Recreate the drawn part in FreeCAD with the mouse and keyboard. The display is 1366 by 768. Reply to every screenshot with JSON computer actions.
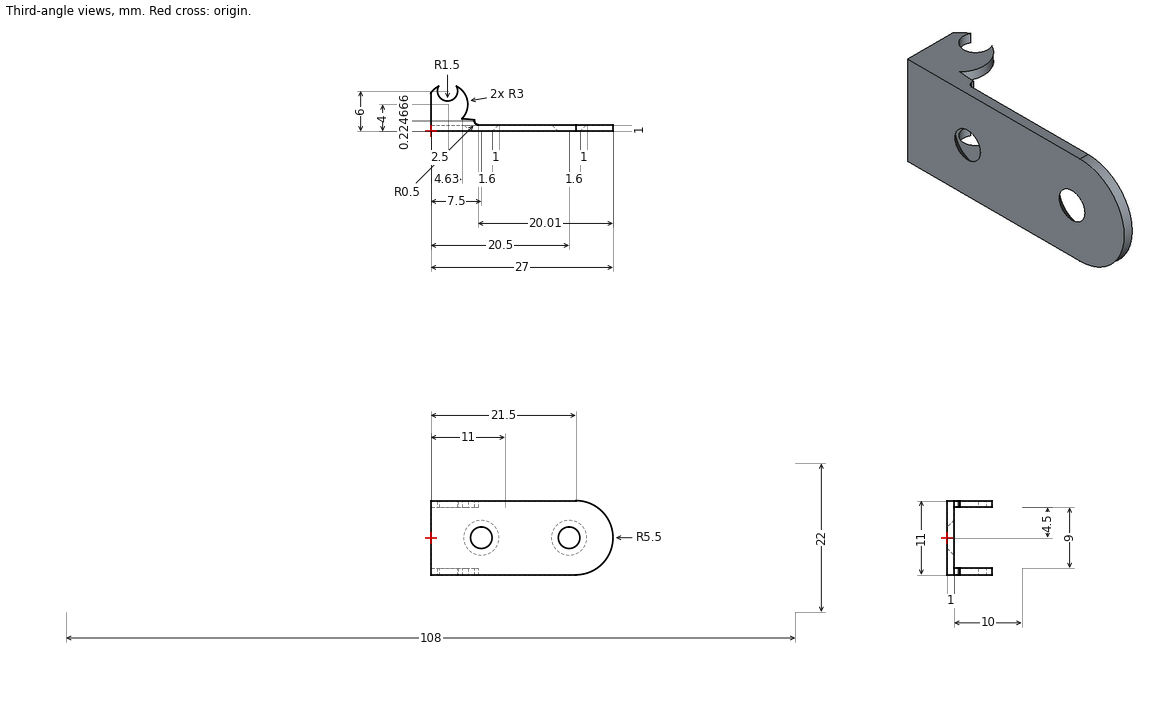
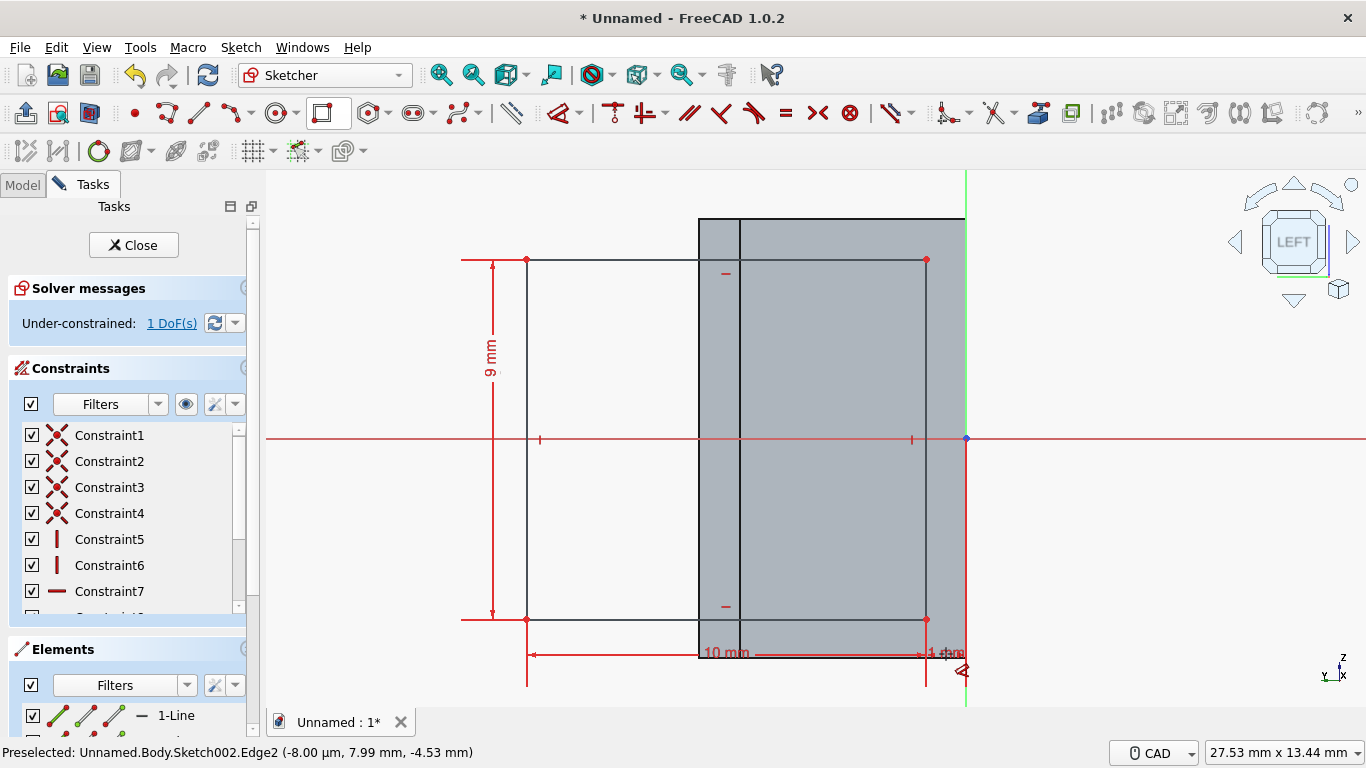
{"action": "left_click", "coordinate": [527, 260]}
{"action": "left_click", "coordinate": [1000, 349]}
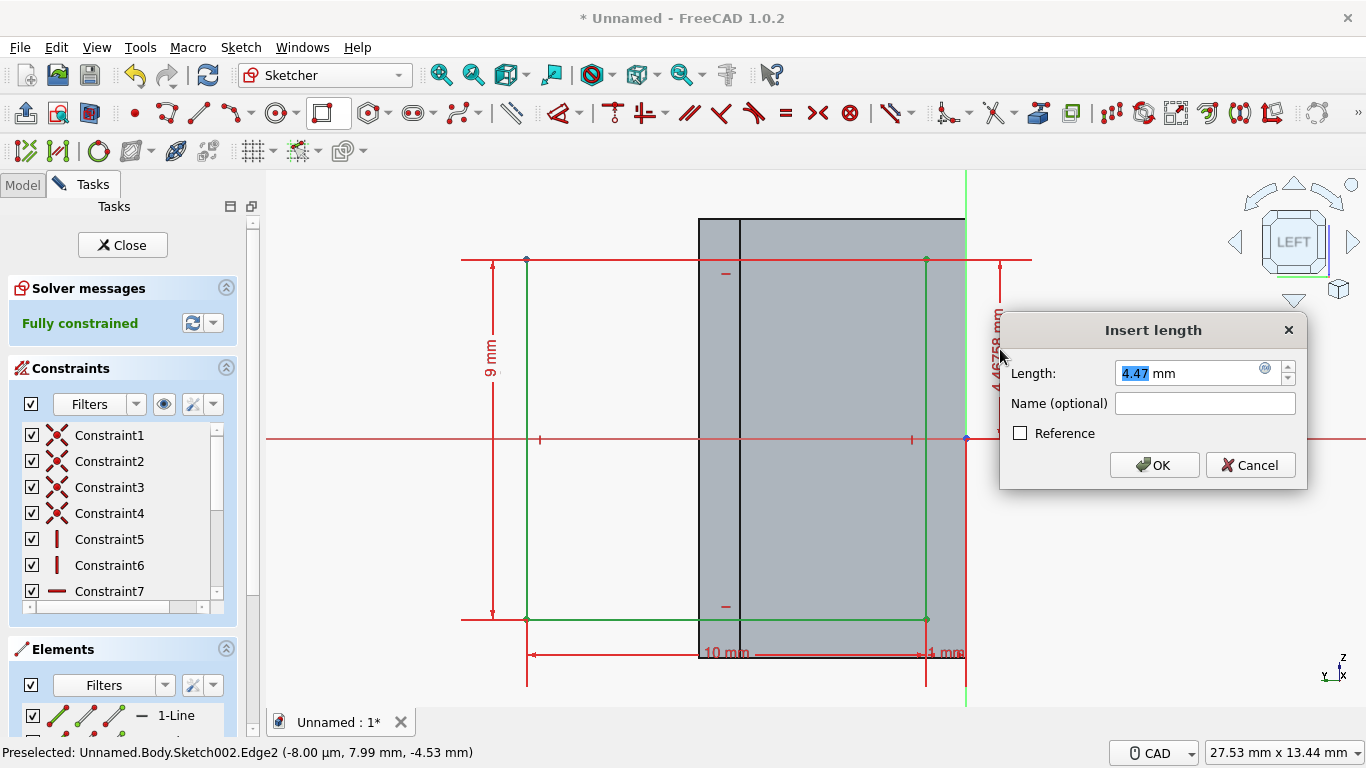
{"action": "type", "text": "4.5"}
{"action": "key", "text": "Return"}
{"action": "key", "text": "Escape"}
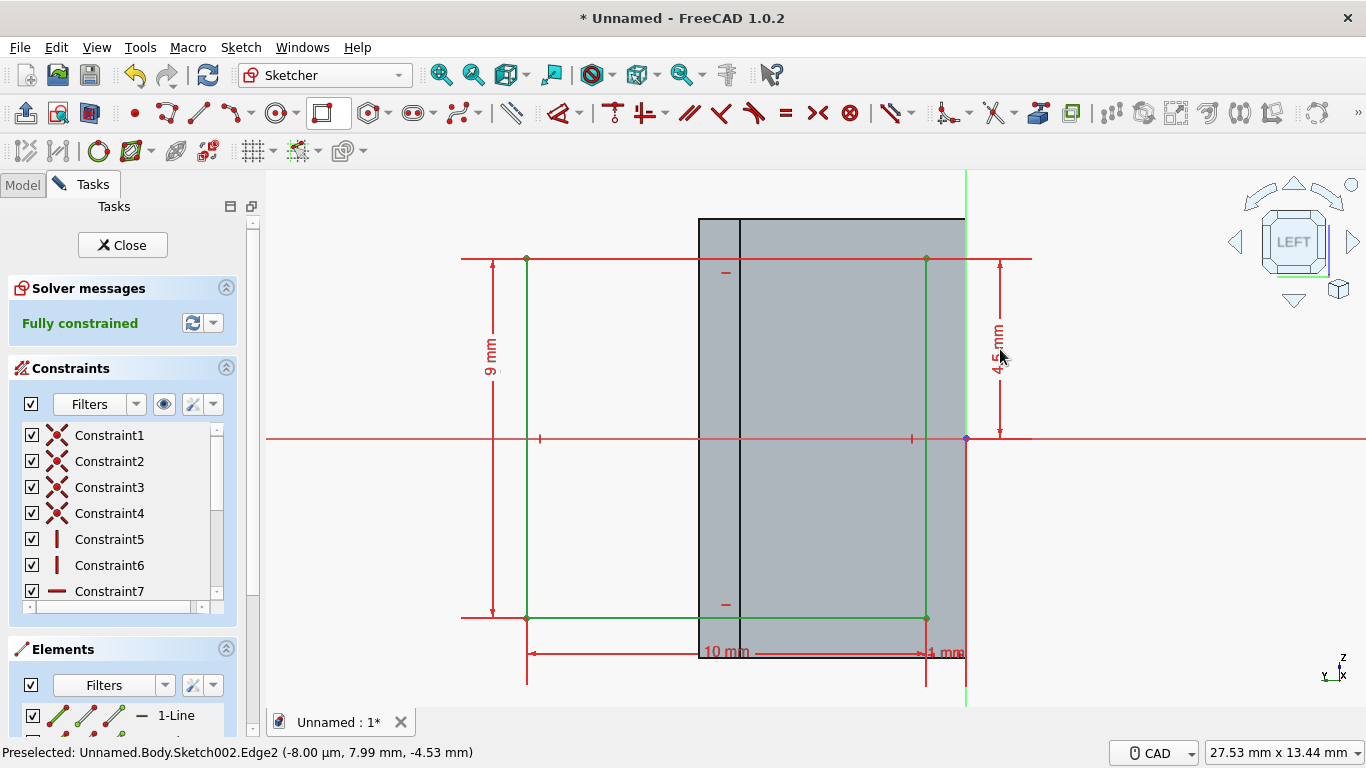
{"action": "left_click", "coordinate": [123, 245]}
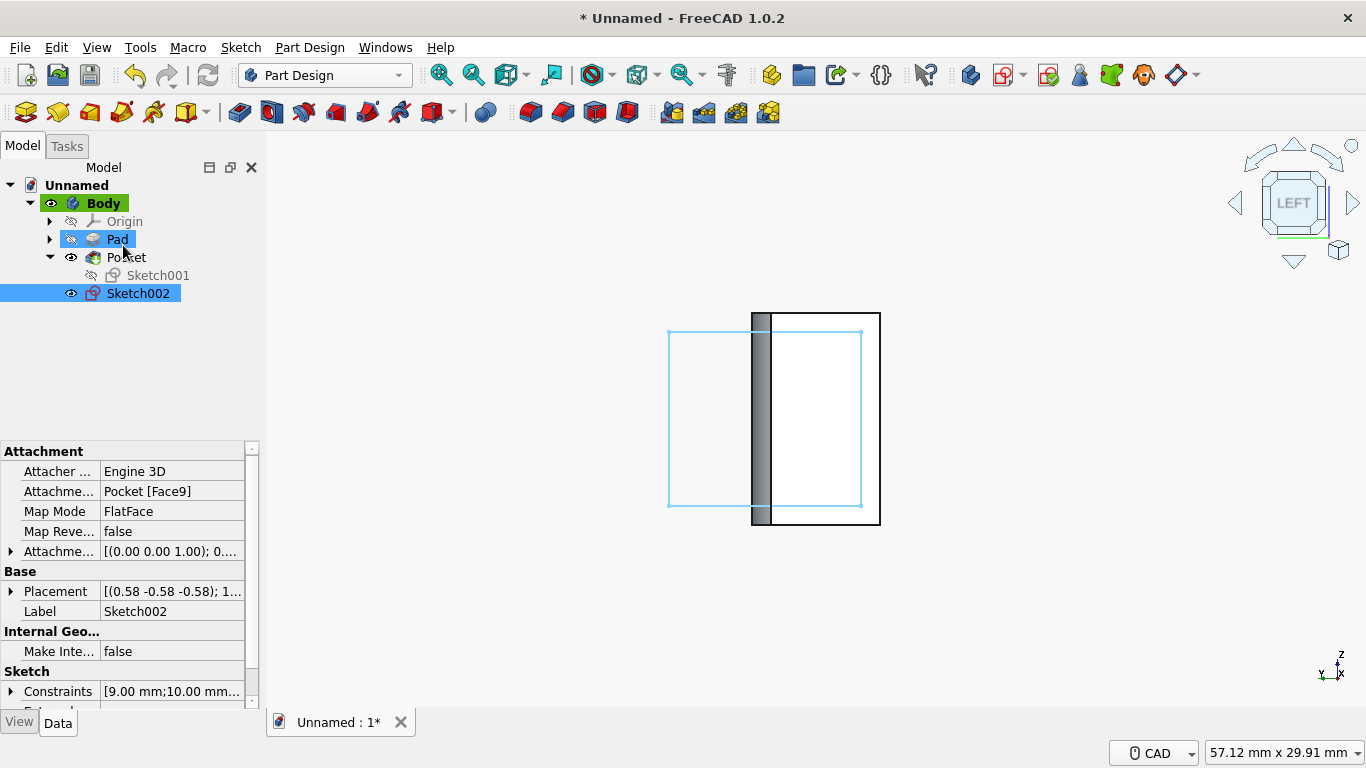
{"action": "left_click", "coordinate": [240, 112]}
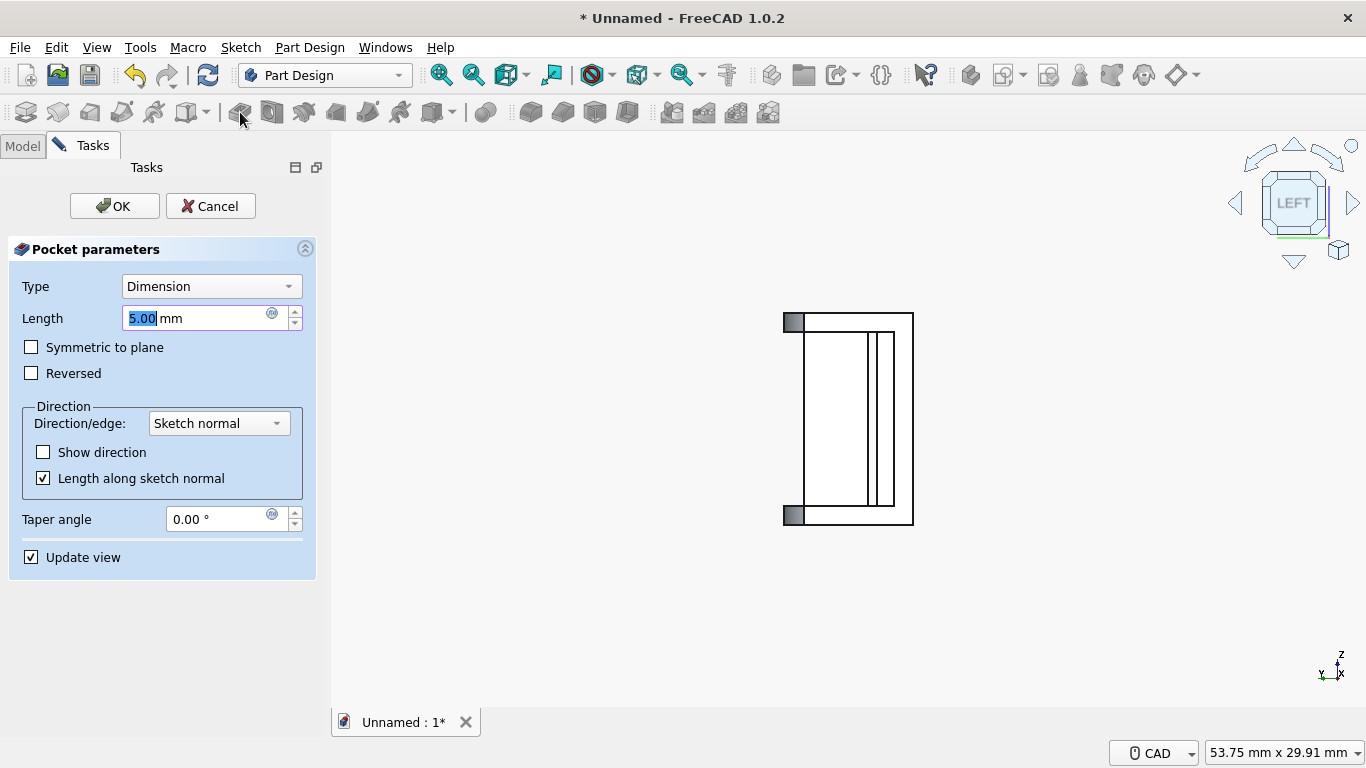
{"action": "type", "text": "11"}
{"action": "key", "text": "Tab"}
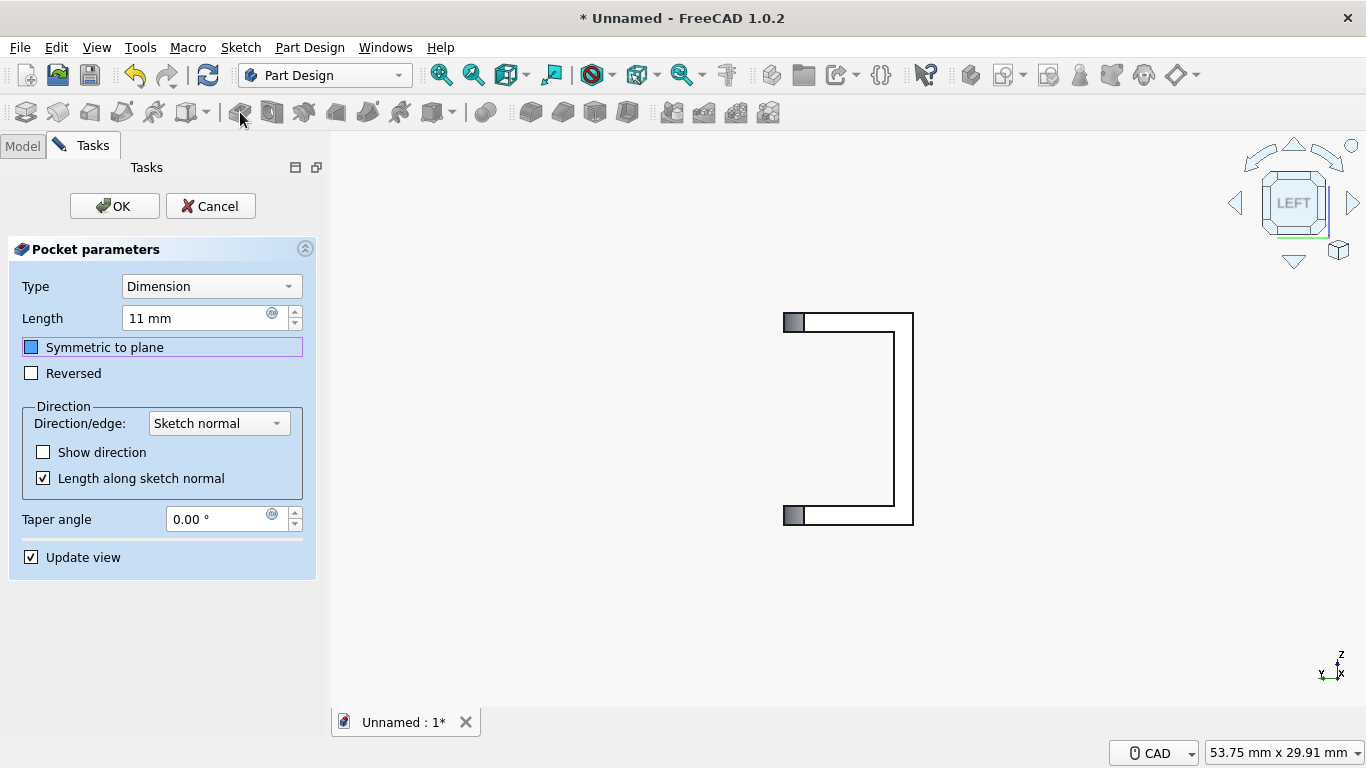
{"action": "left_click", "coordinate": [115, 206]}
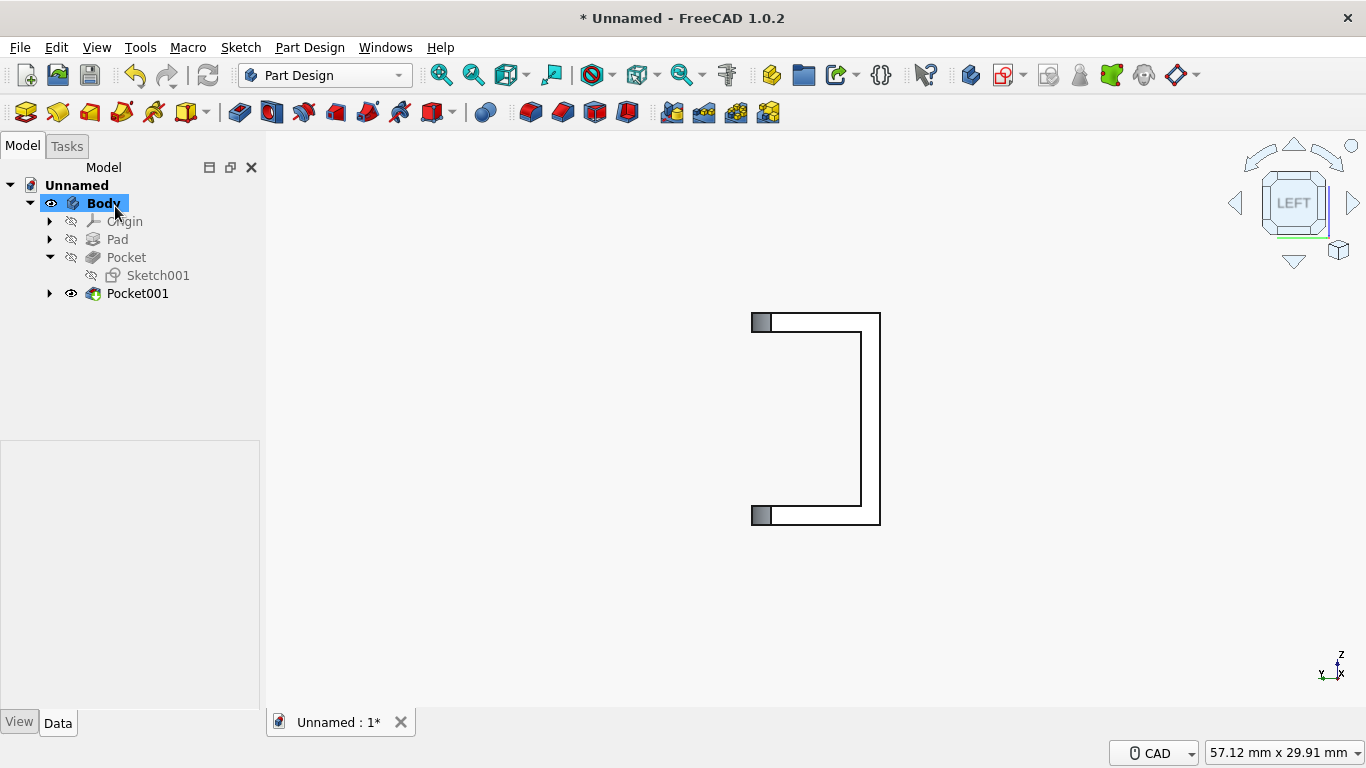
{"action": "left_click", "coordinate": [442, 76]}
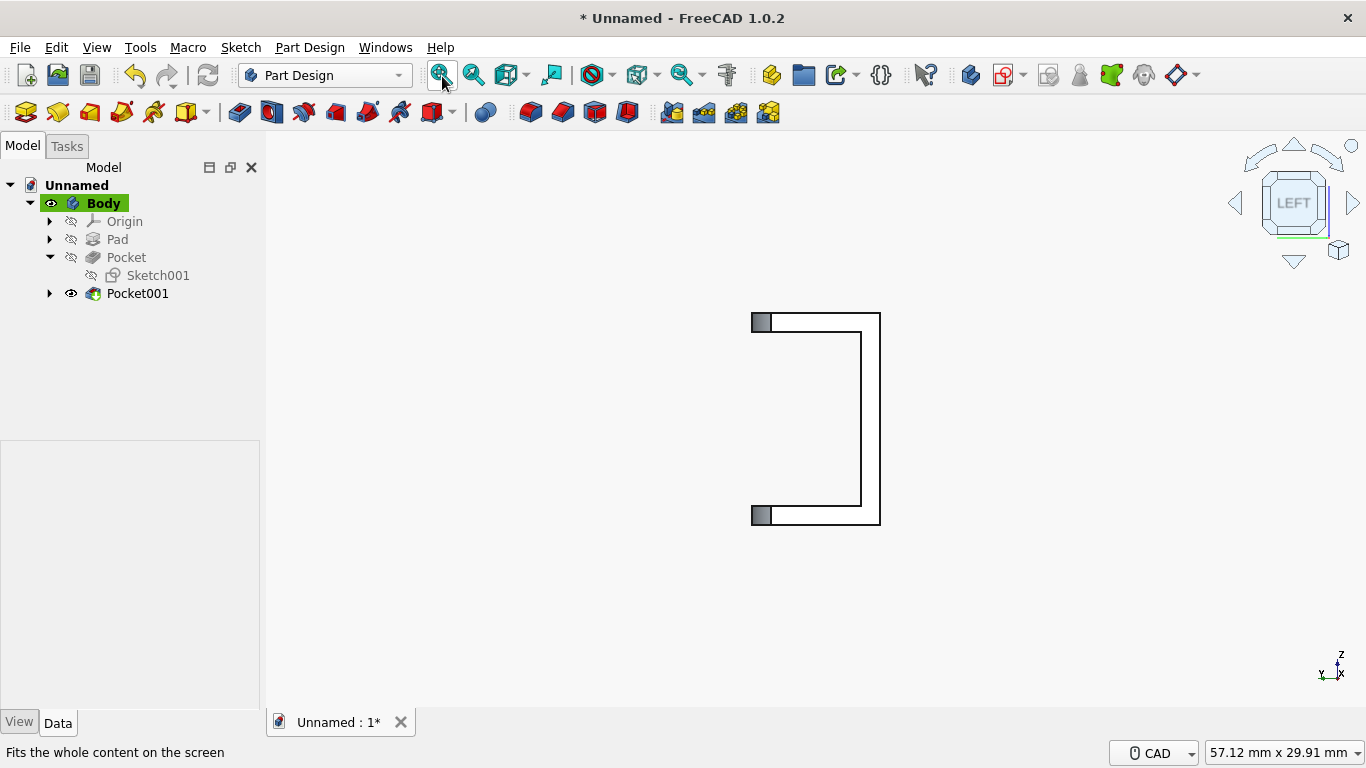
{"action": "left_click", "coordinate": [1004, 76]}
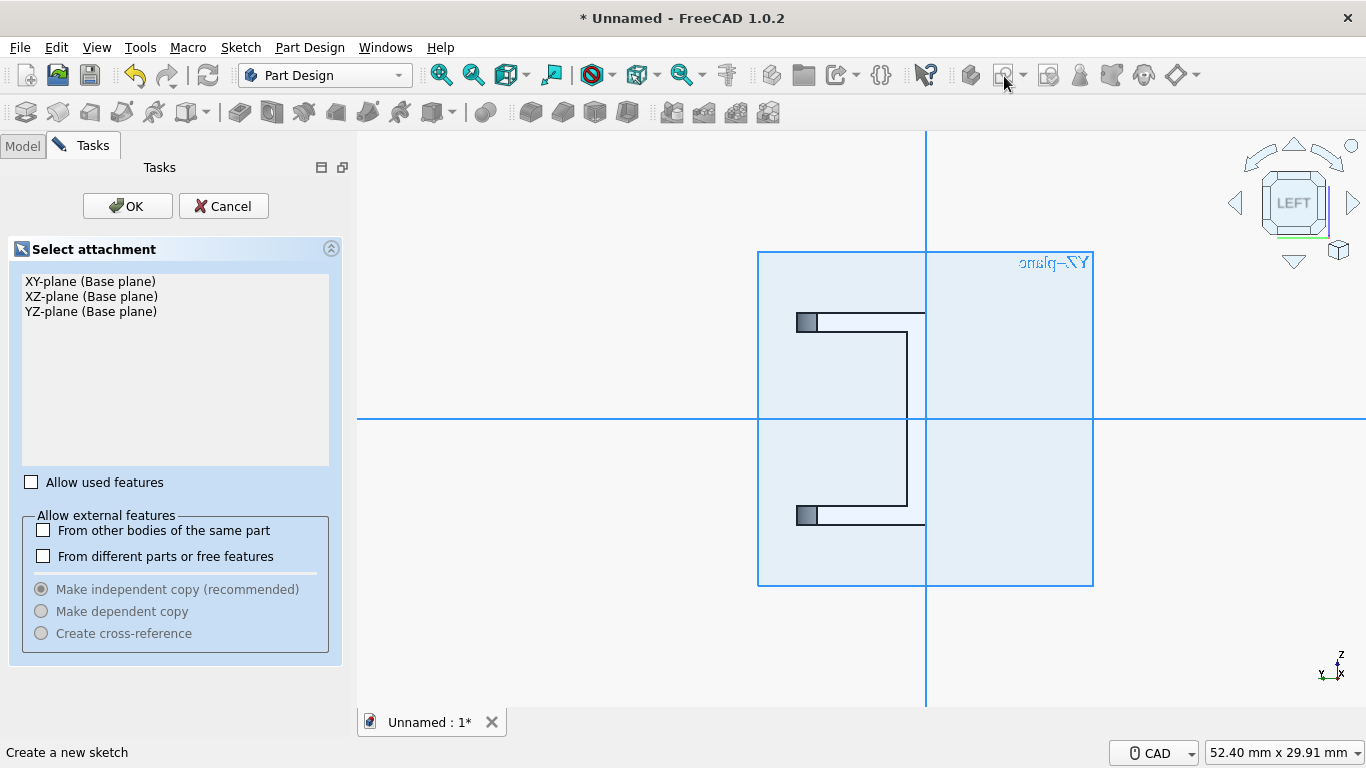
{"action": "left_click", "coordinate": [82, 282]}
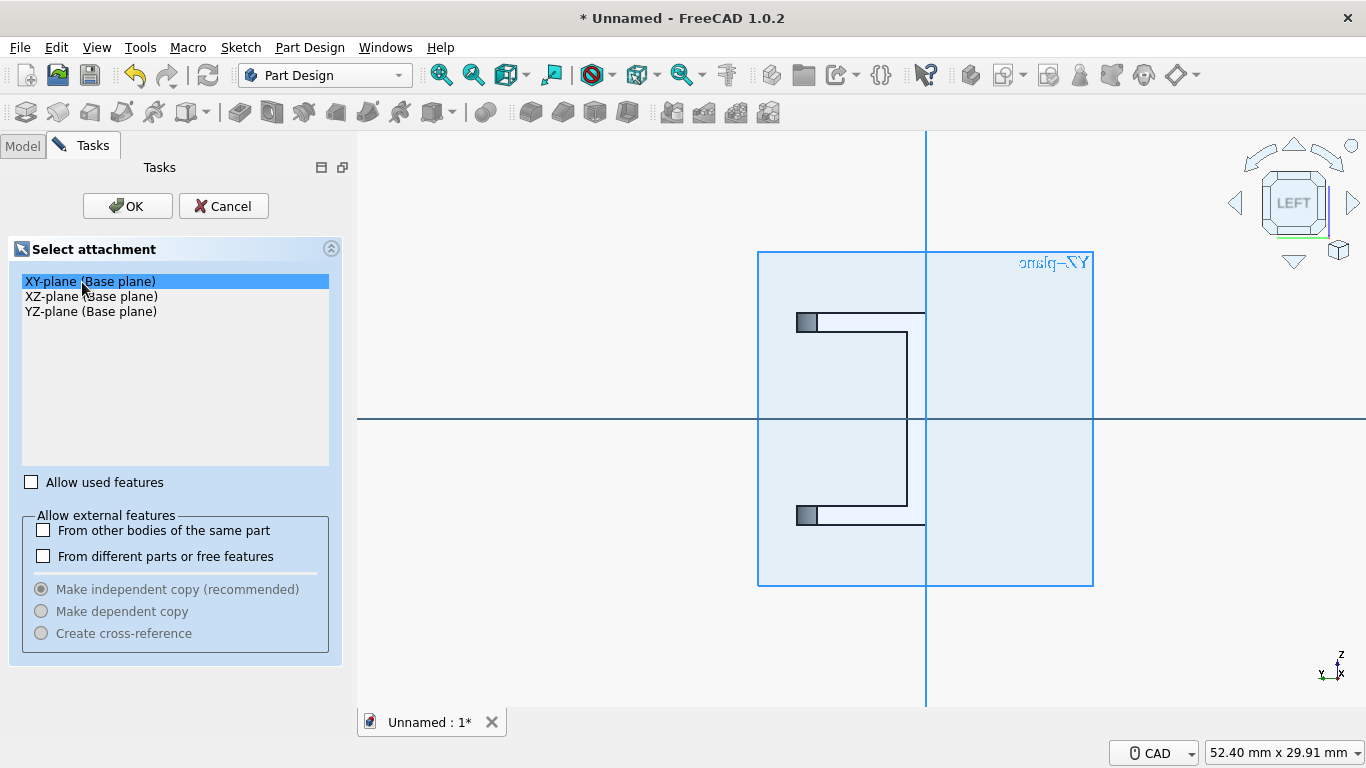
{"action": "left_click", "coordinate": [128, 206]}